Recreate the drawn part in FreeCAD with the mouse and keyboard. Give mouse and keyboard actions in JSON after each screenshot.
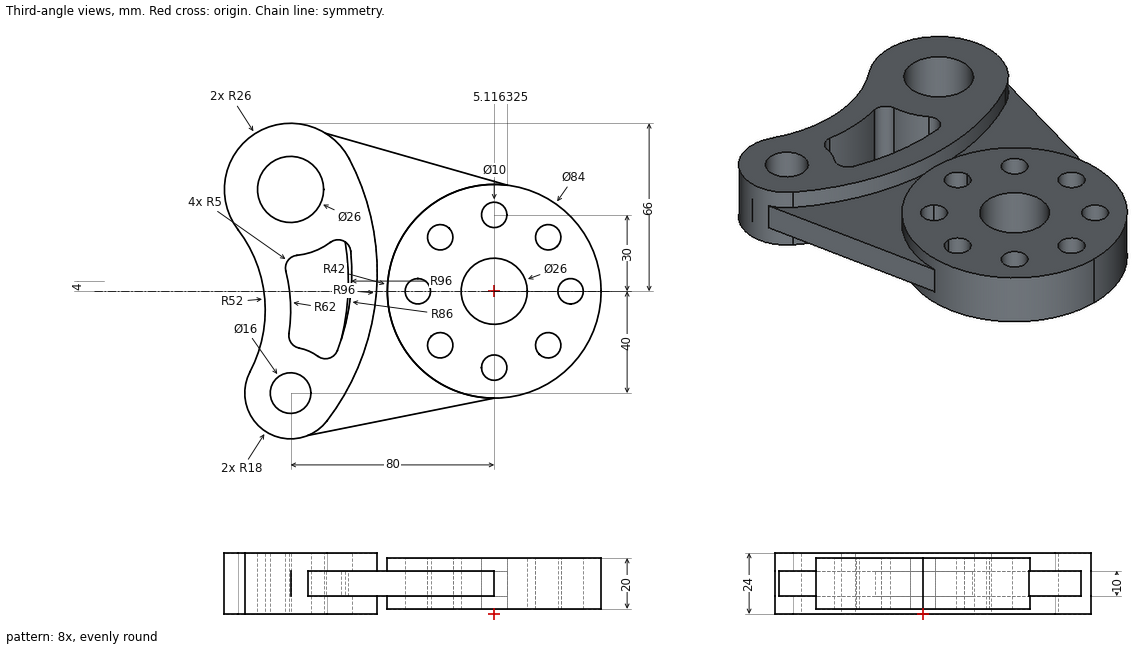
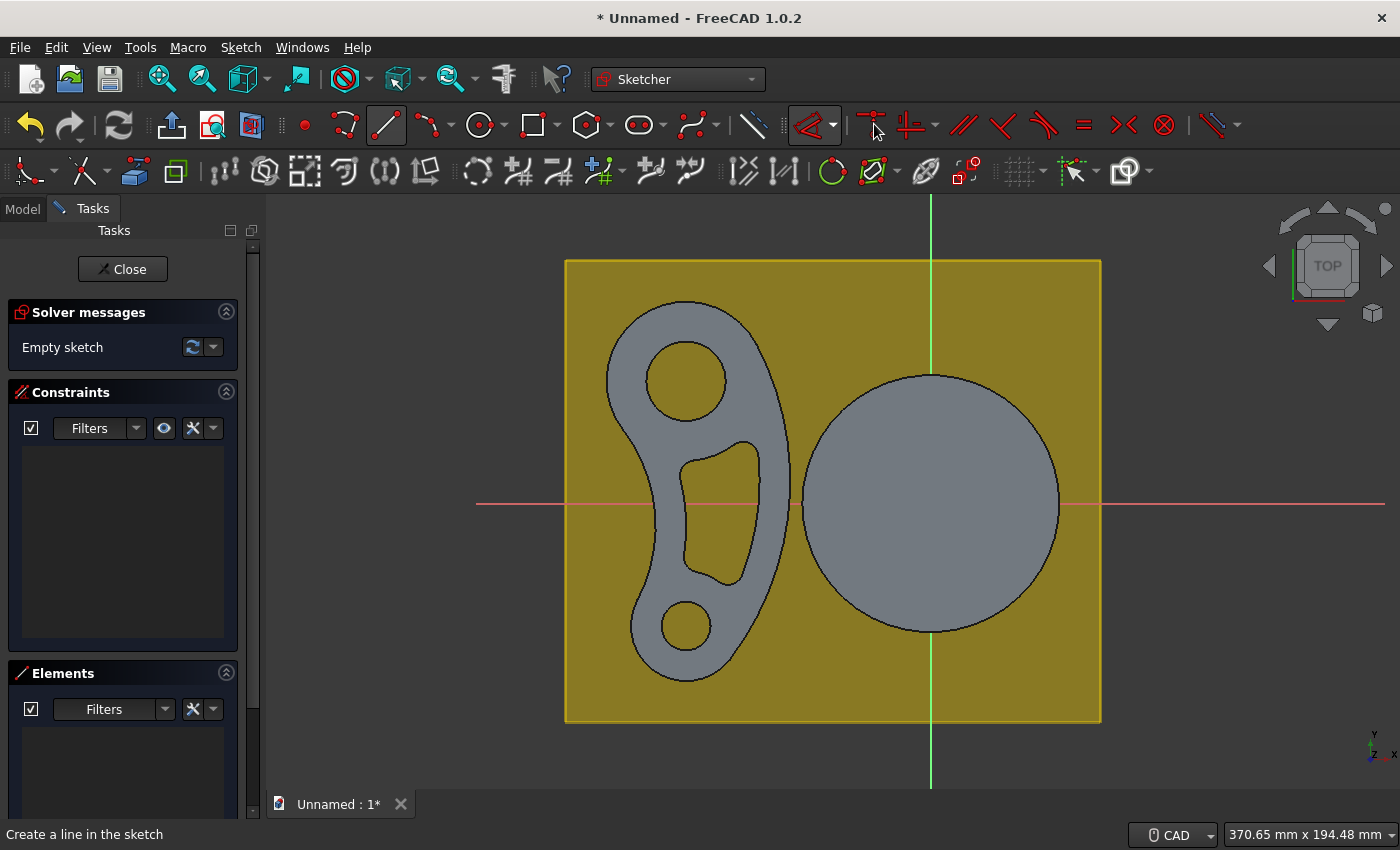
{"action": "left_click", "coordinate": [252, 126]}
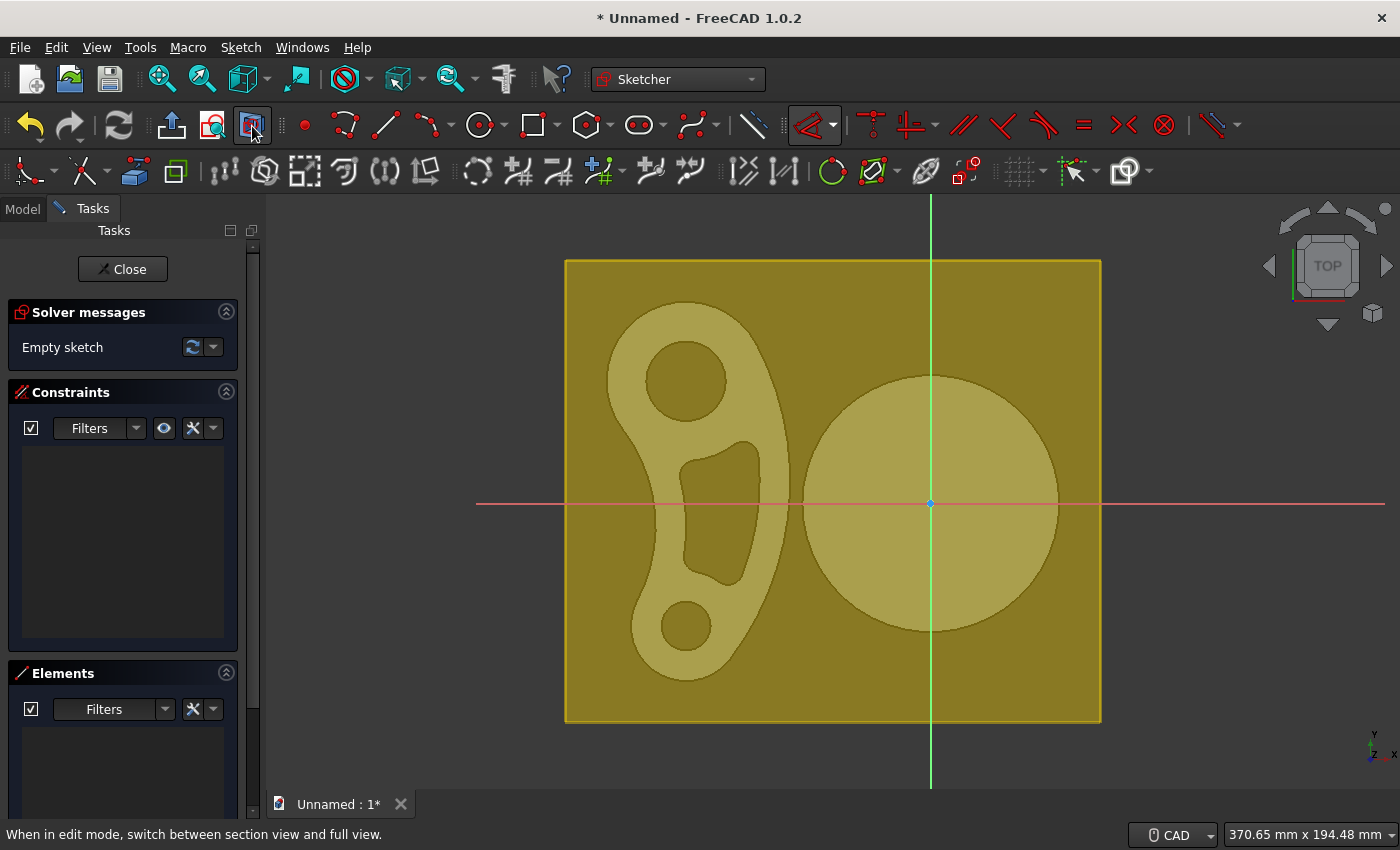
{"action": "left_click", "coordinate": [386, 126]}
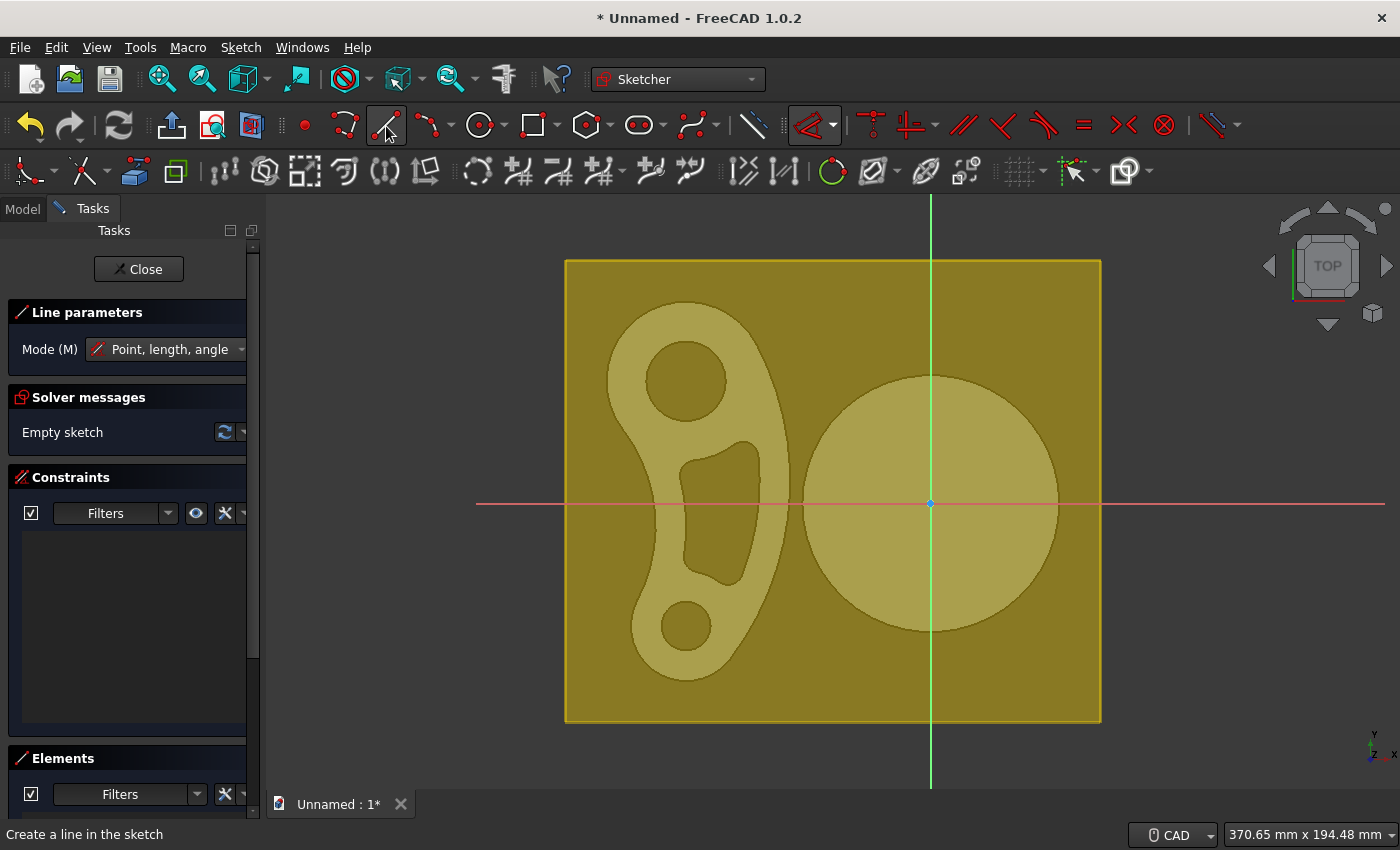
{"action": "left_click", "coordinate": [946, 376]}
{"action": "left_click", "coordinate": [686, 302]}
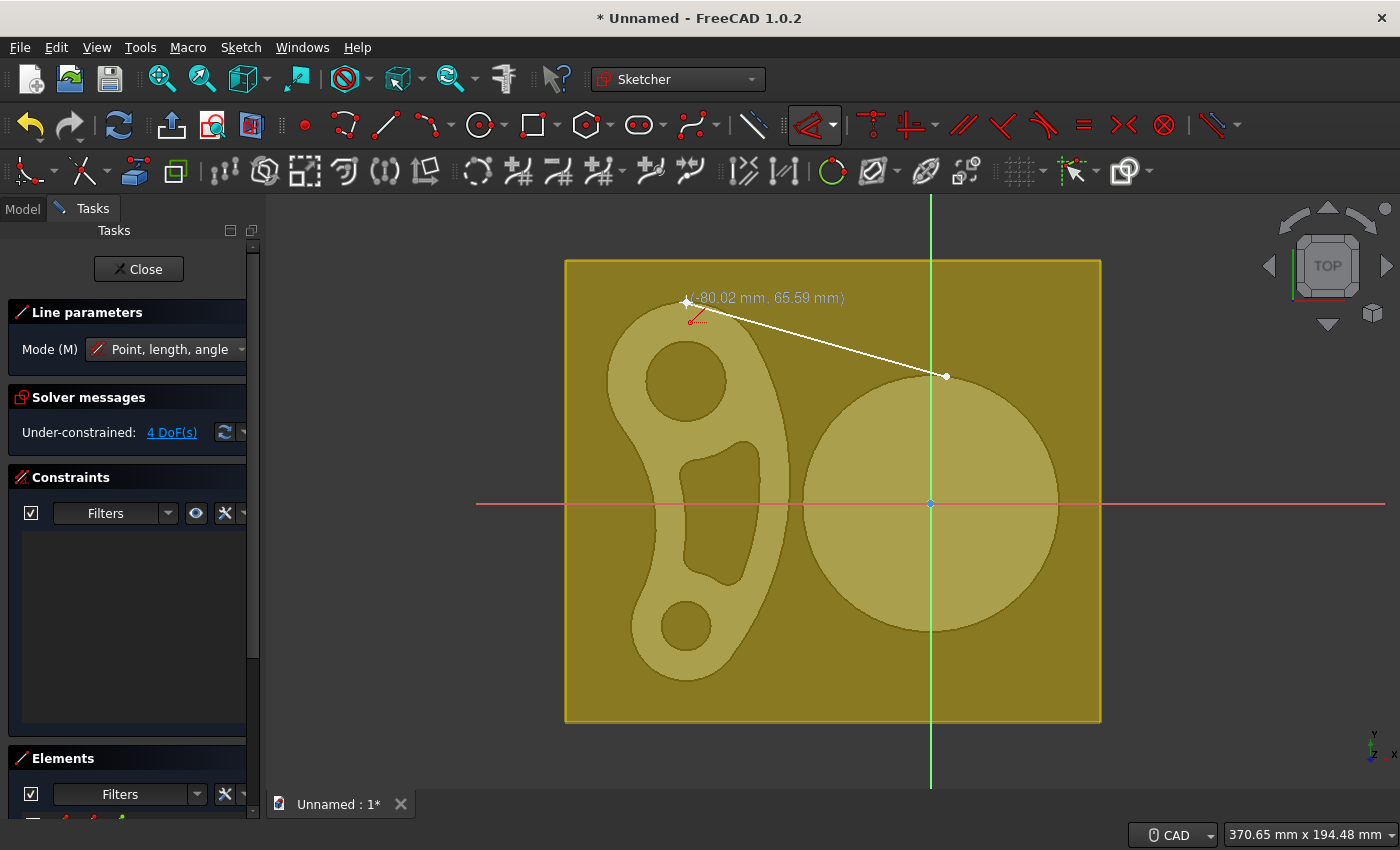
{"action": "left_click", "coordinate": [686, 681]}
{"action": "left_click", "coordinate": [931, 632]}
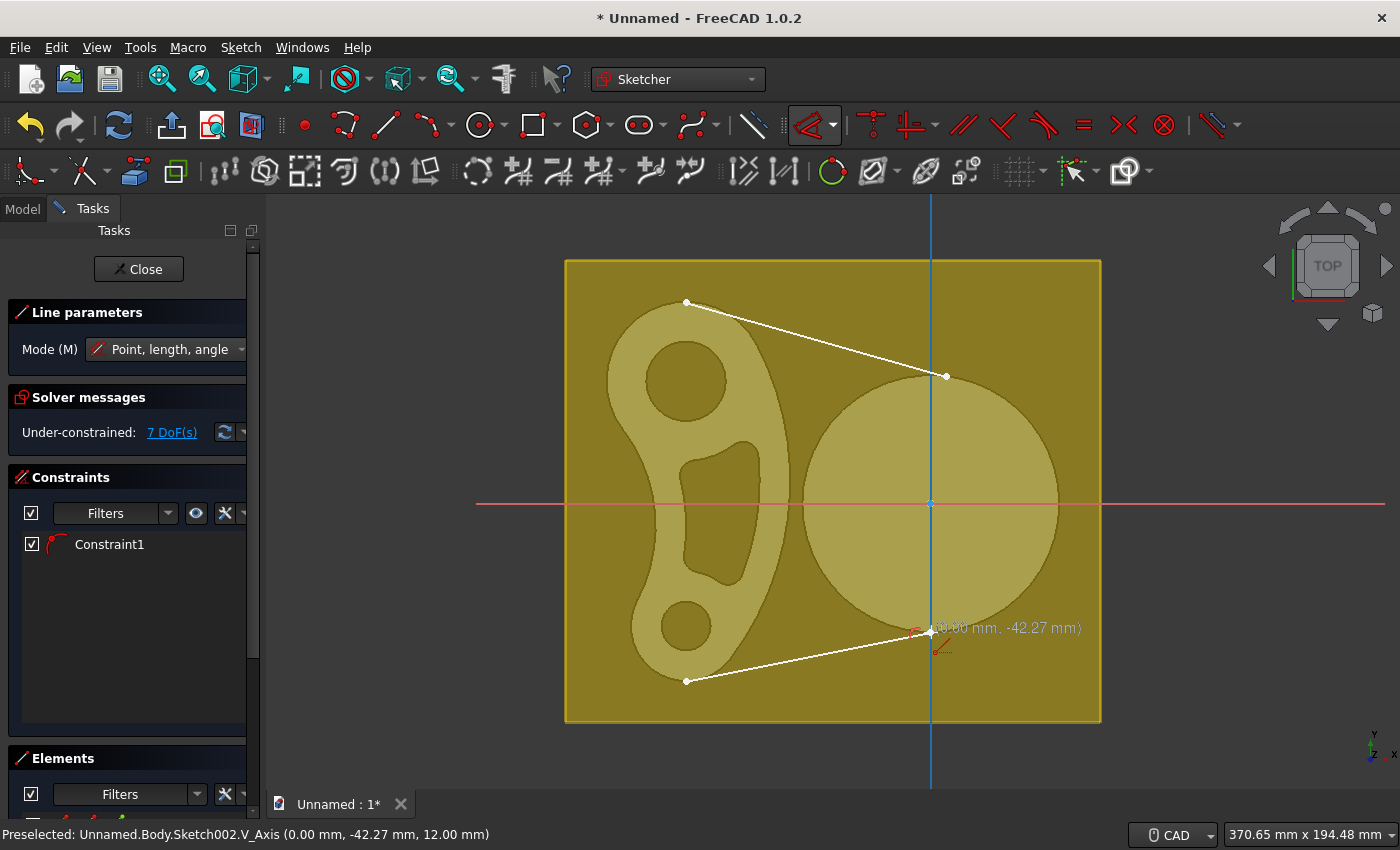
{"action": "left_click", "coordinate": [428, 126]}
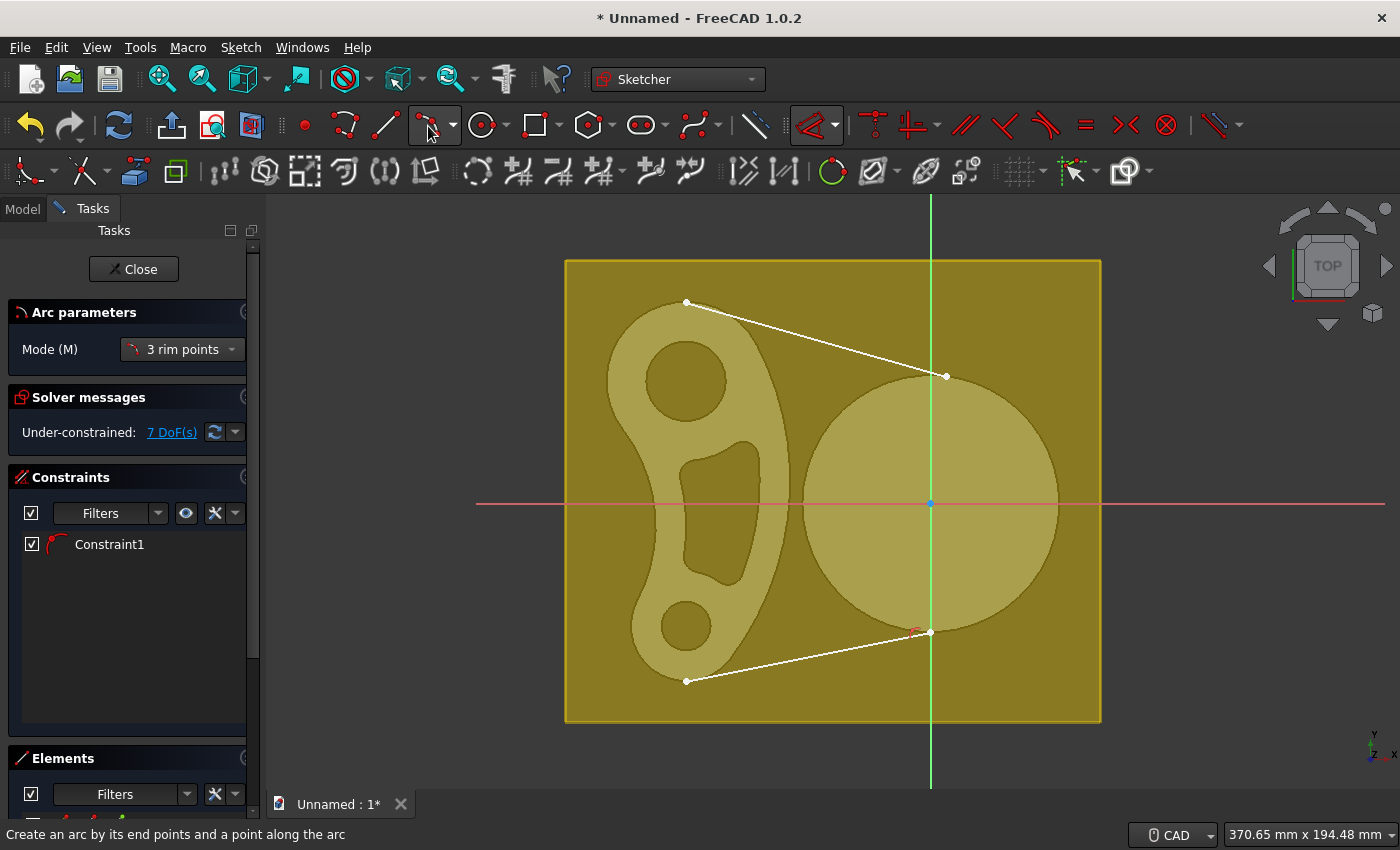
{"action": "left_click", "coordinate": [686, 303]}
{"action": "left_click", "coordinate": [686, 682]}
{"action": "left_click", "coordinate": [753, 533]}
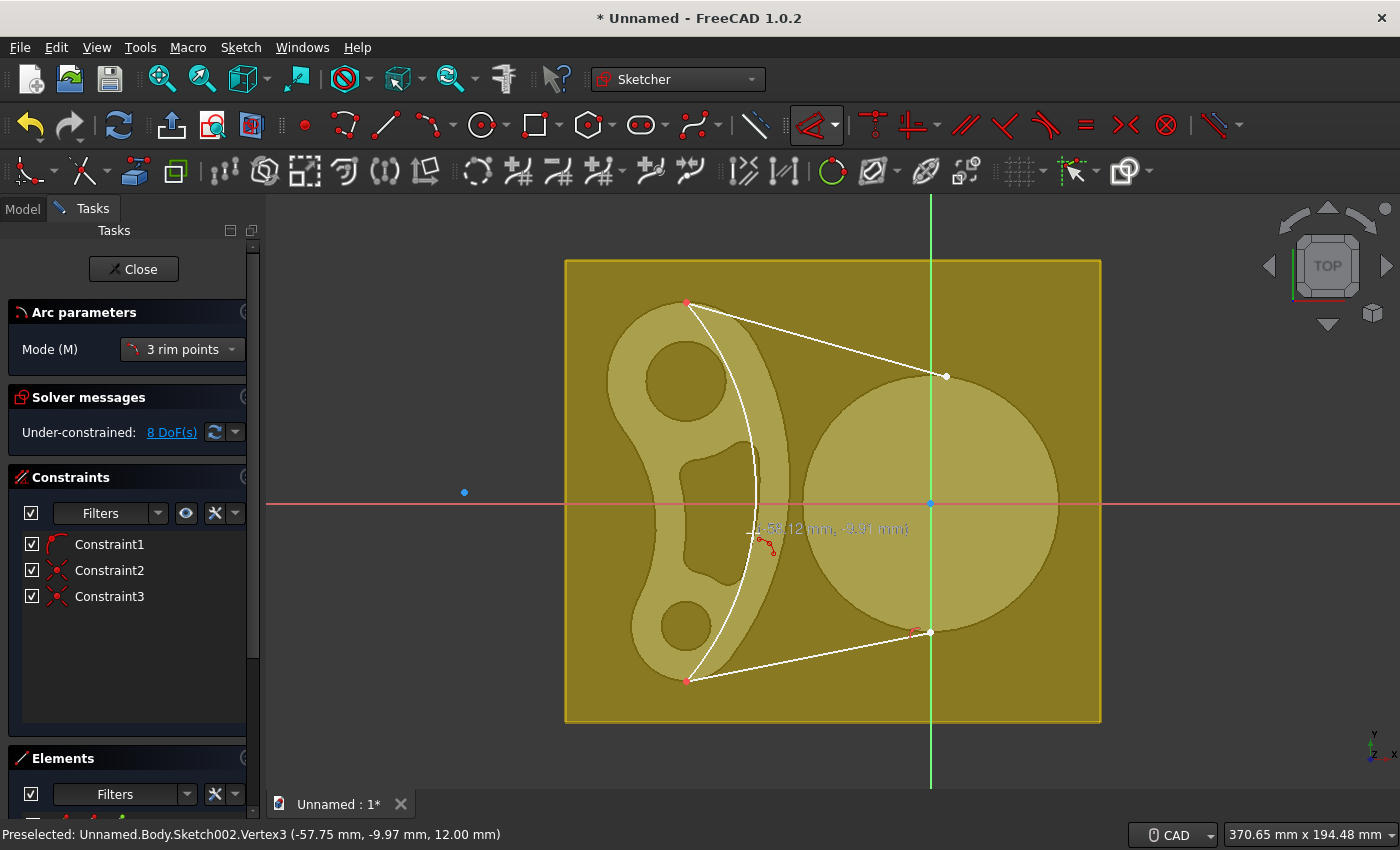
{"action": "left_click", "coordinate": [931, 633]}
{"action": "left_click", "coordinate": [946, 377]}
{"action": "left_click", "coordinate": [812, 455]}
{"action": "key", "text": "Escape"}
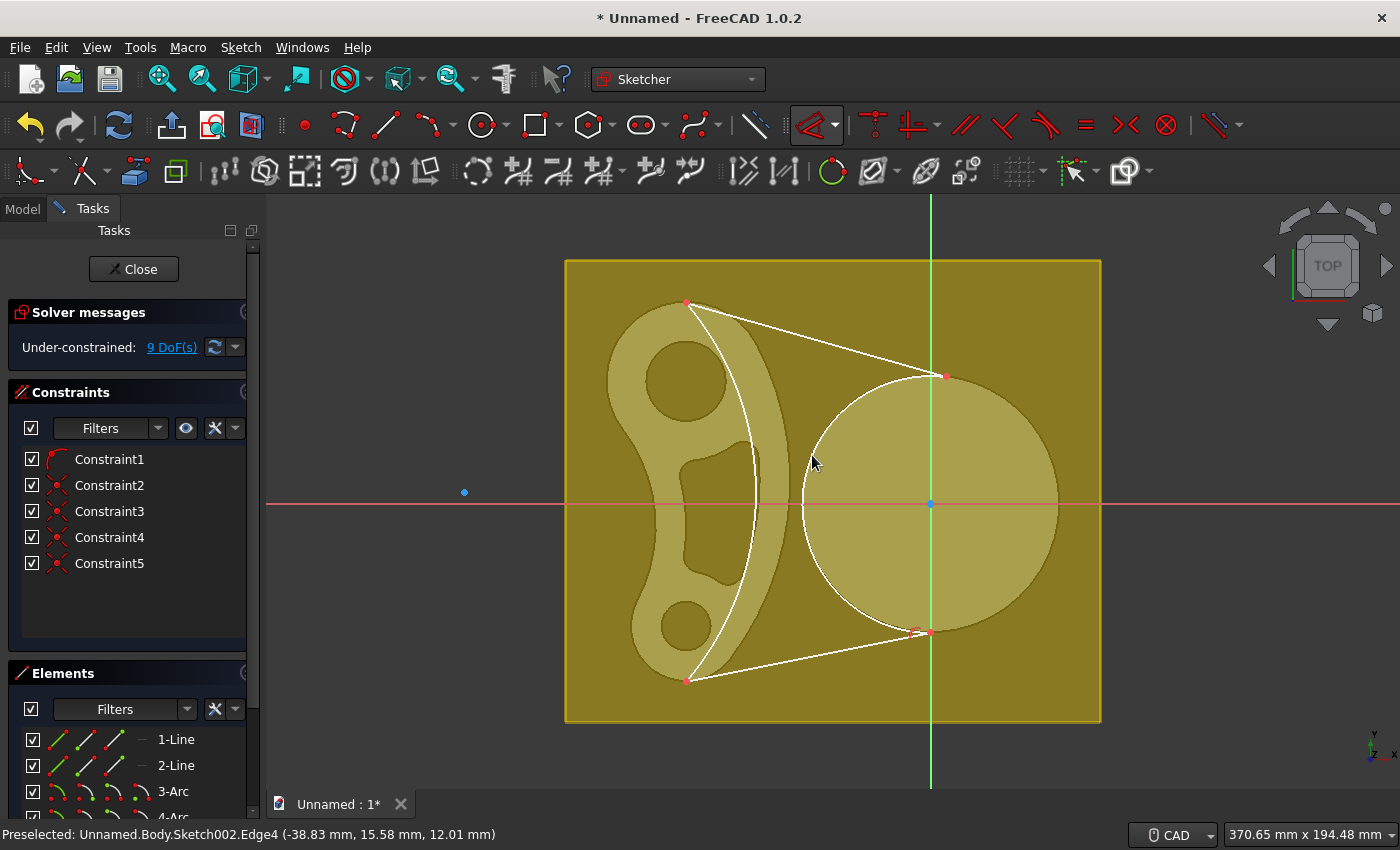
{"action": "left_click_drag", "start_coordinate": [921, 494], "coordinate": [941, 515]}